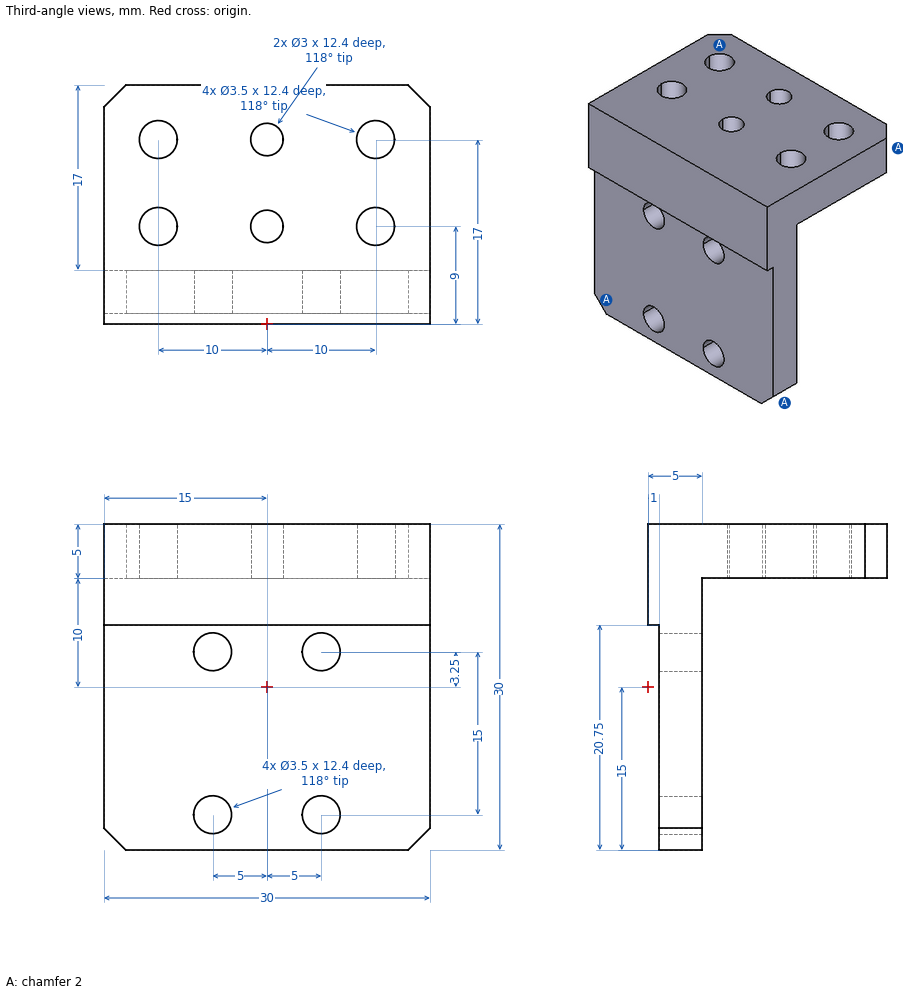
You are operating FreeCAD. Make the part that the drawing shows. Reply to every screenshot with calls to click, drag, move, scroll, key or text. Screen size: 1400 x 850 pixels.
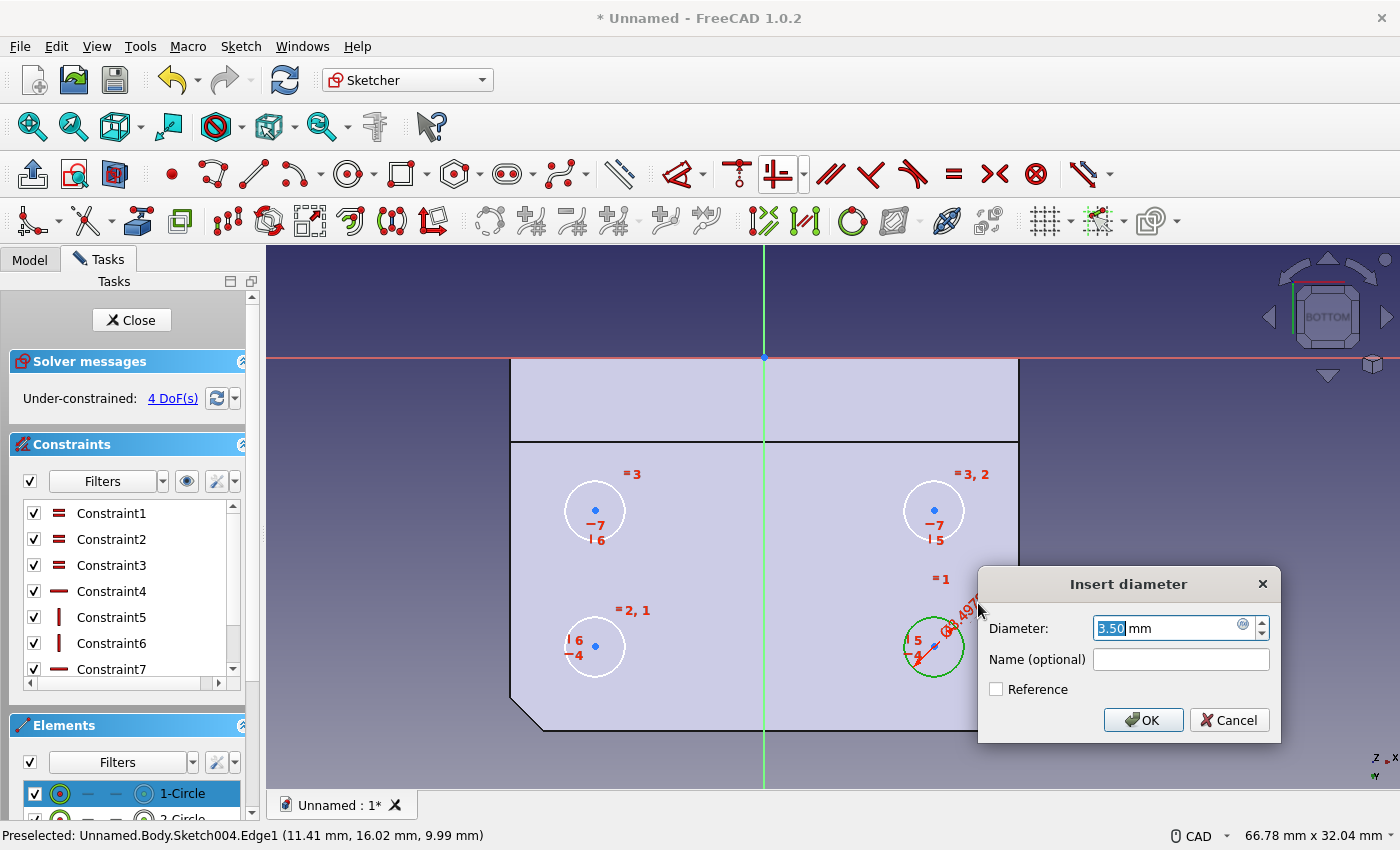
text(3.5)
key(Return)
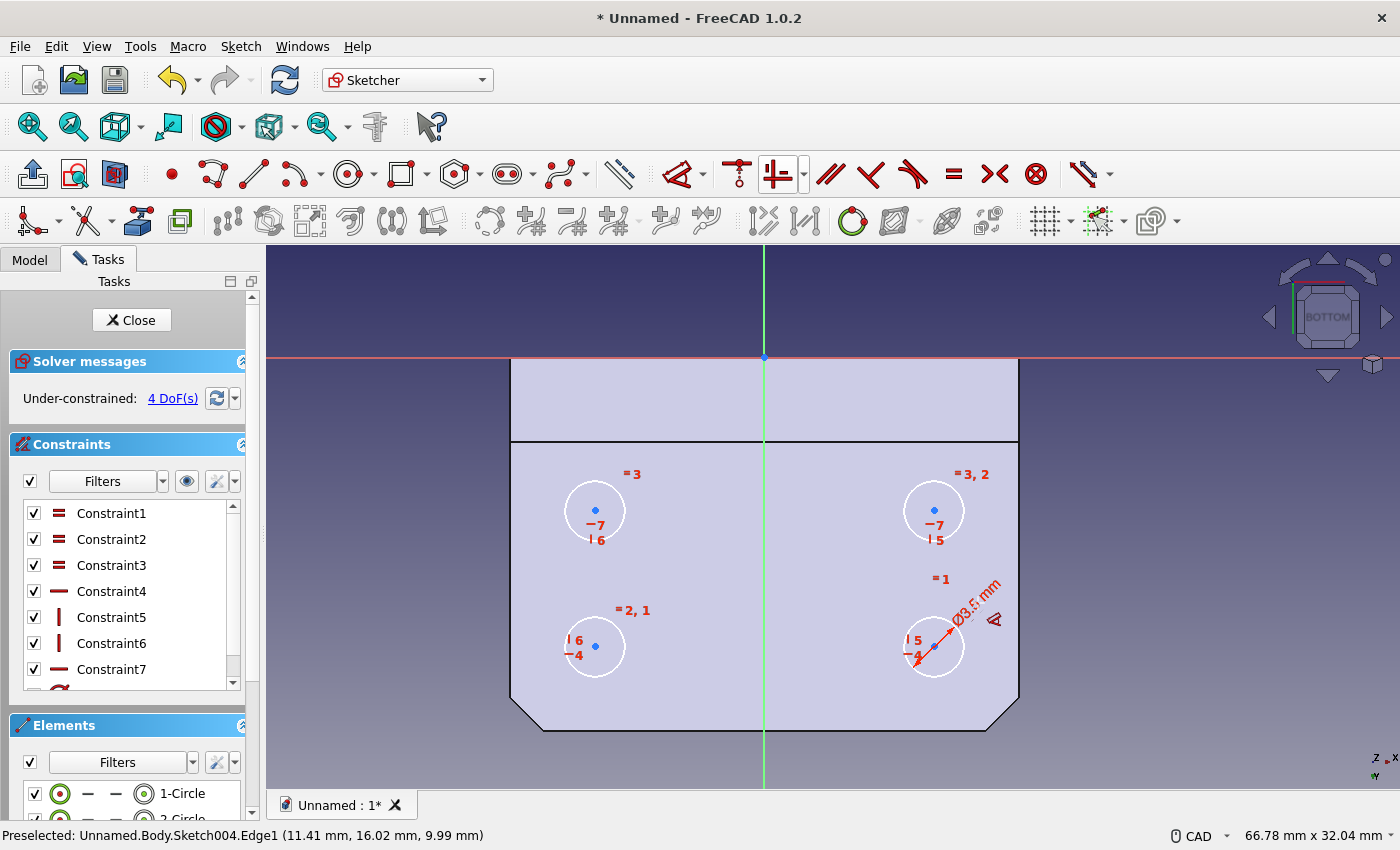
click(934, 511)
click(968, 434)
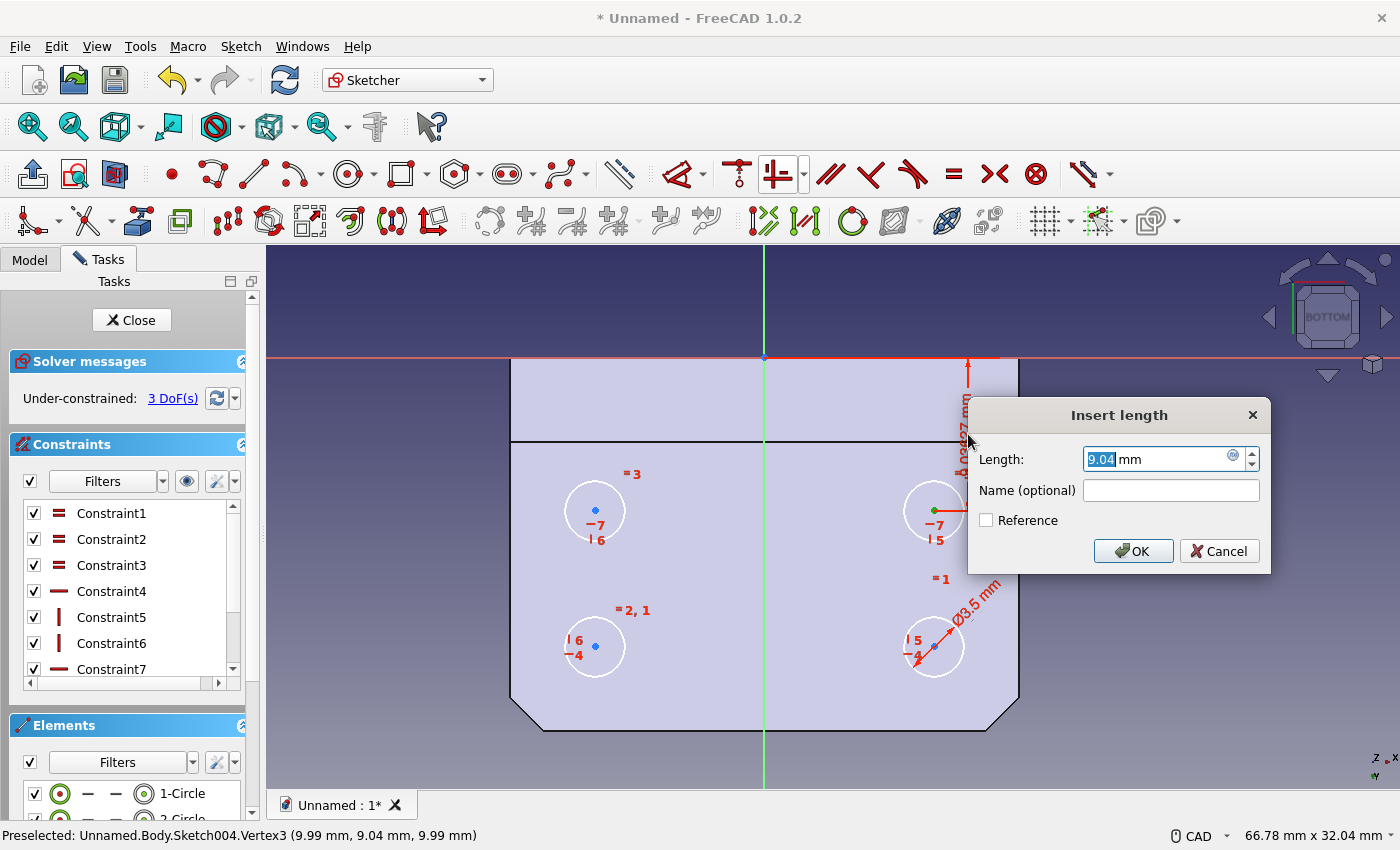
text(9)
key(Return)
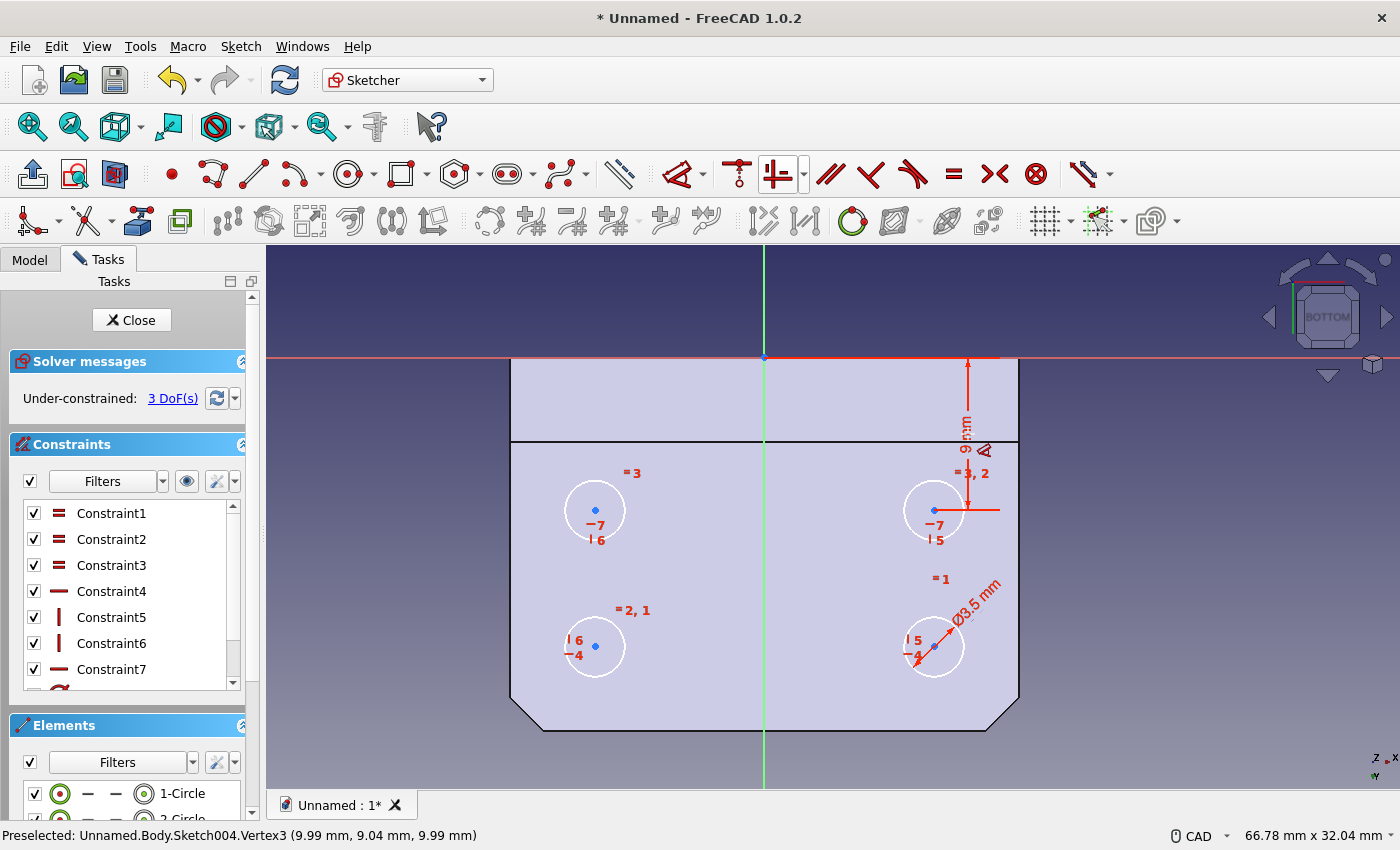
click(934, 647)
click(849, 324)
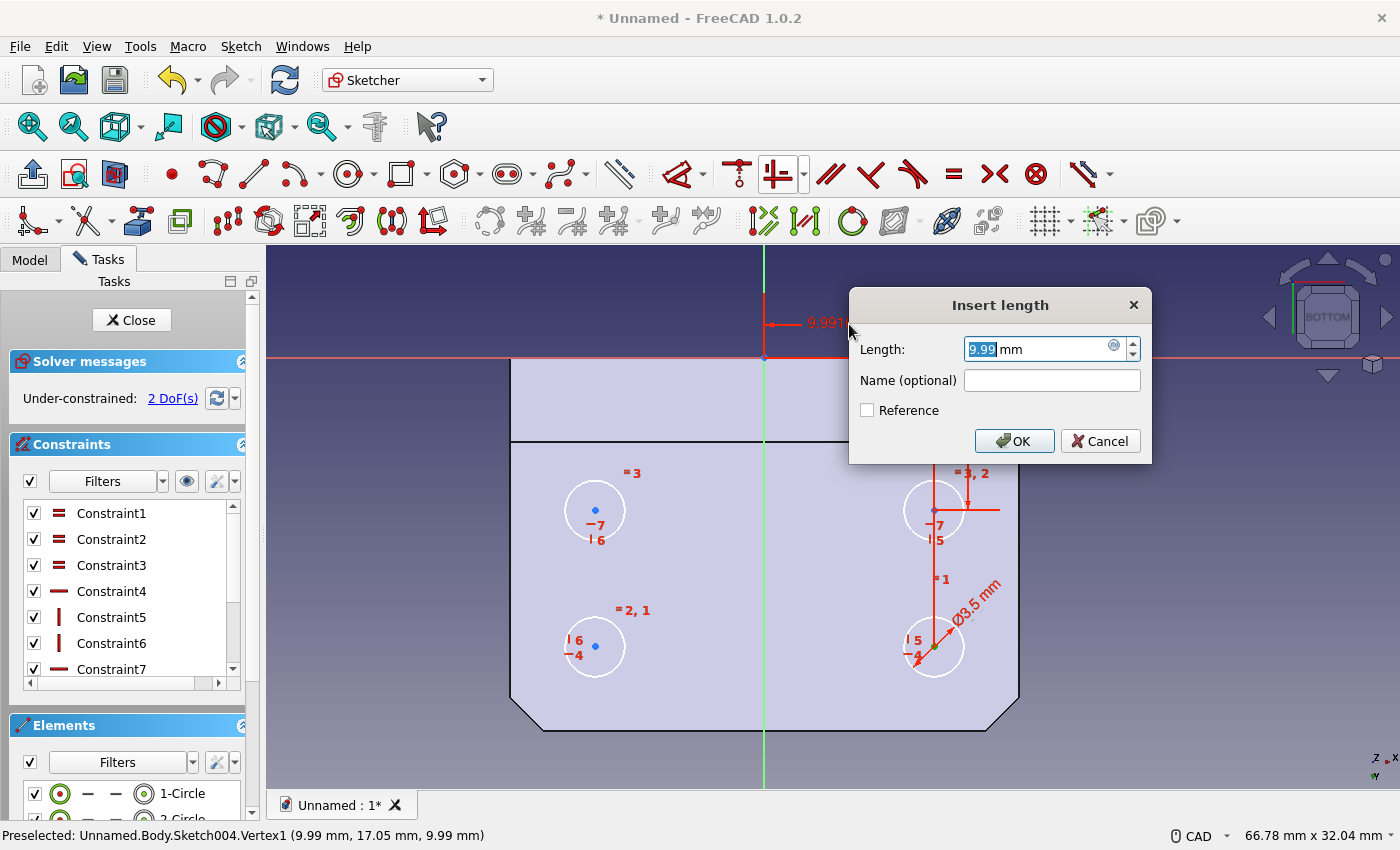
text(10)
key(Return)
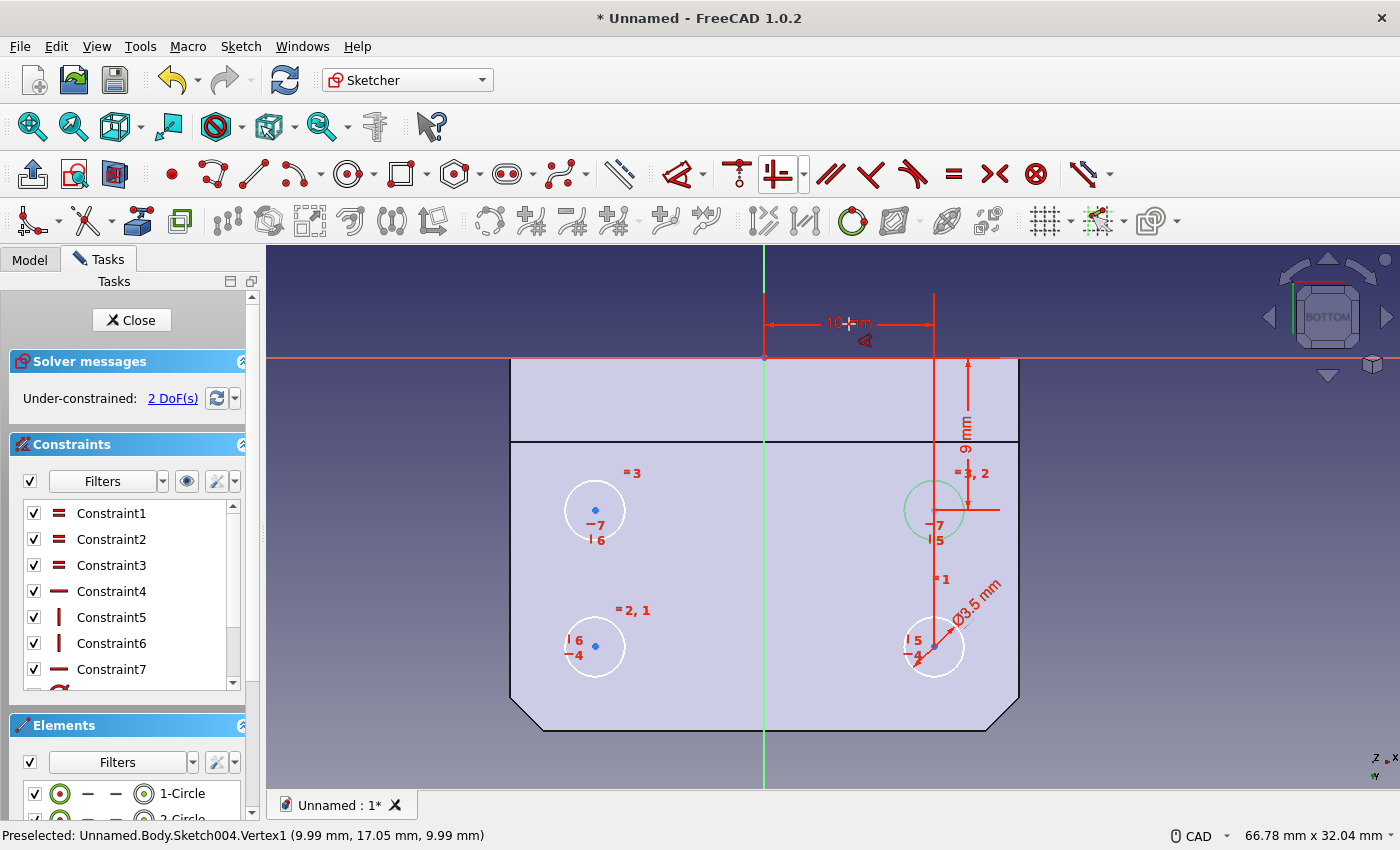
click(934, 647)
click(968, 569)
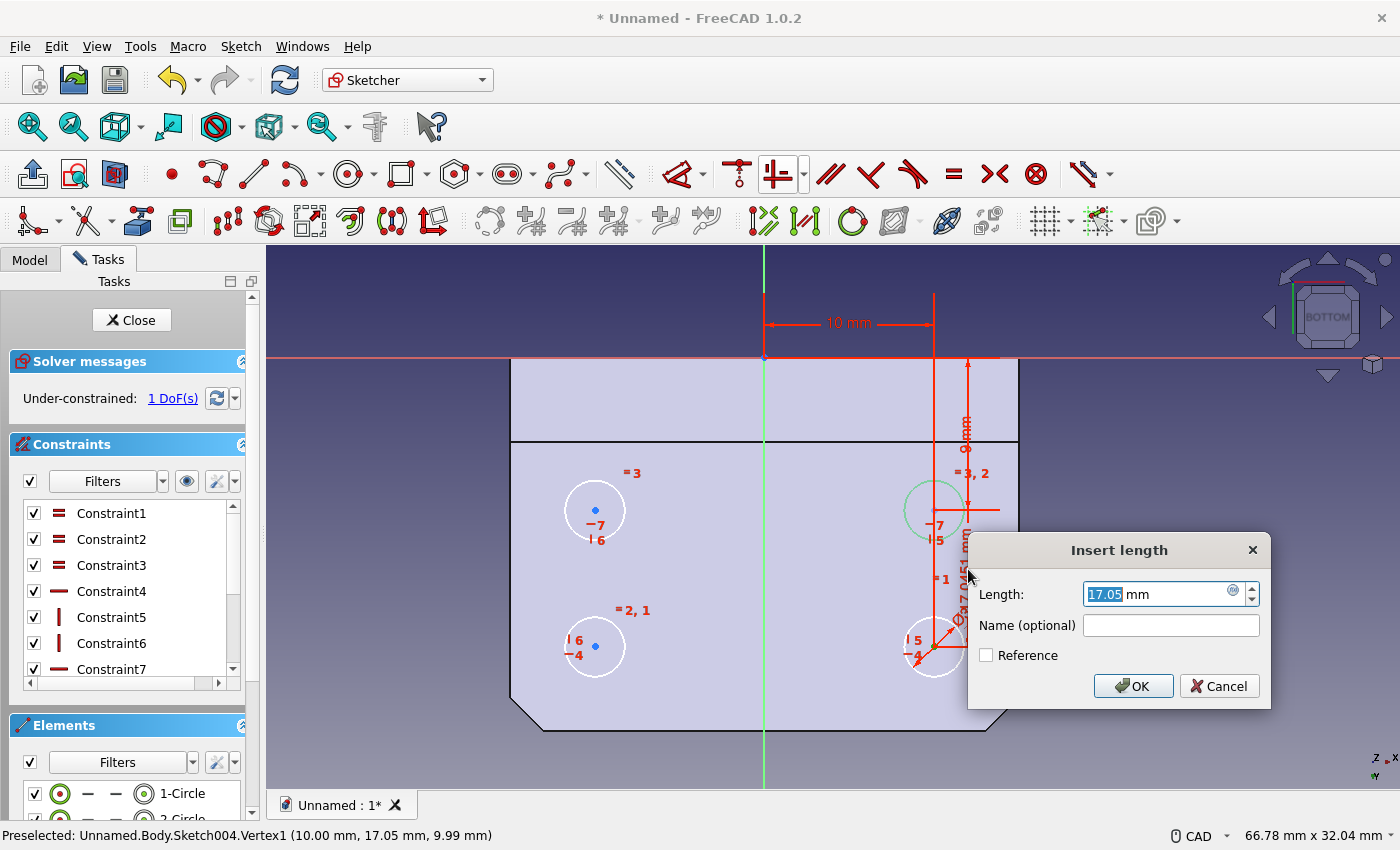
text(17)
key(Return)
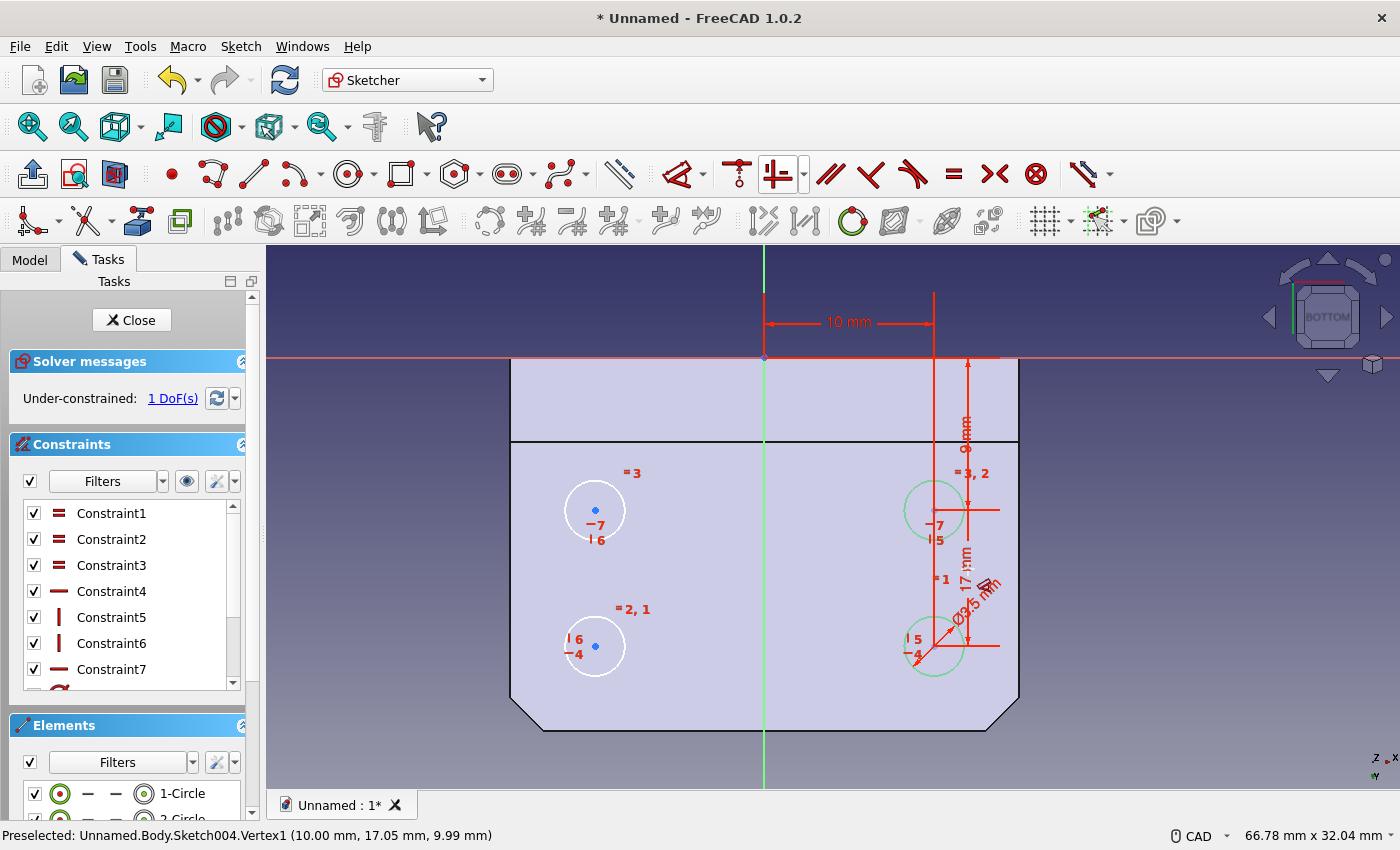
click(595, 646)
click(680, 324)